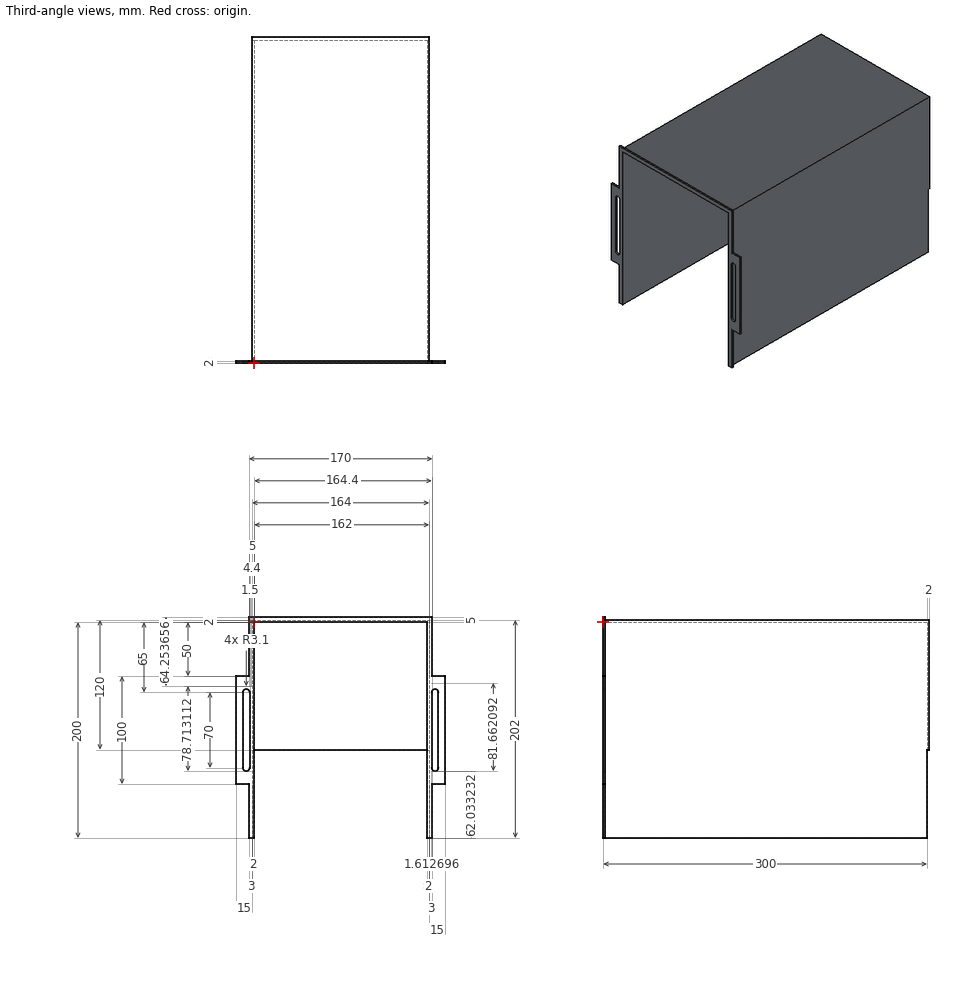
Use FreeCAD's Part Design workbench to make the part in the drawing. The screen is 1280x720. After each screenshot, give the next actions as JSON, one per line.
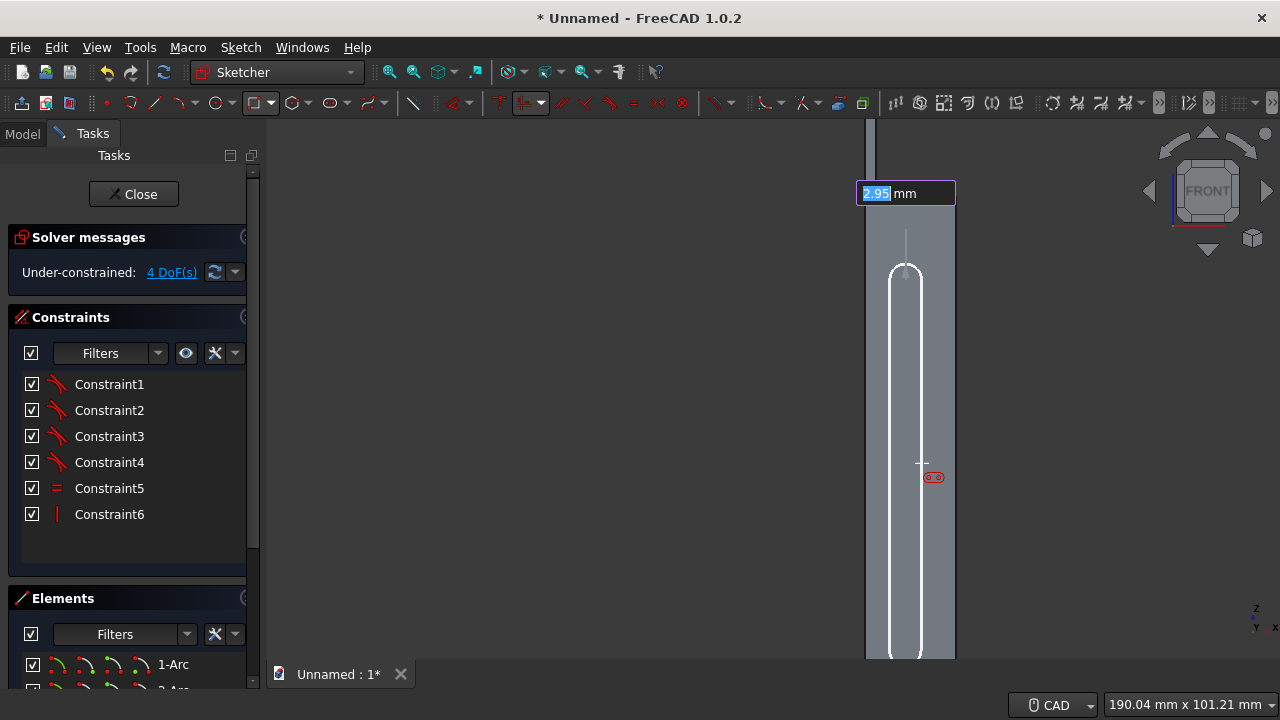
{"action": "left_click", "coordinate": [922, 463]}
{"action": "key", "text": "Escape"}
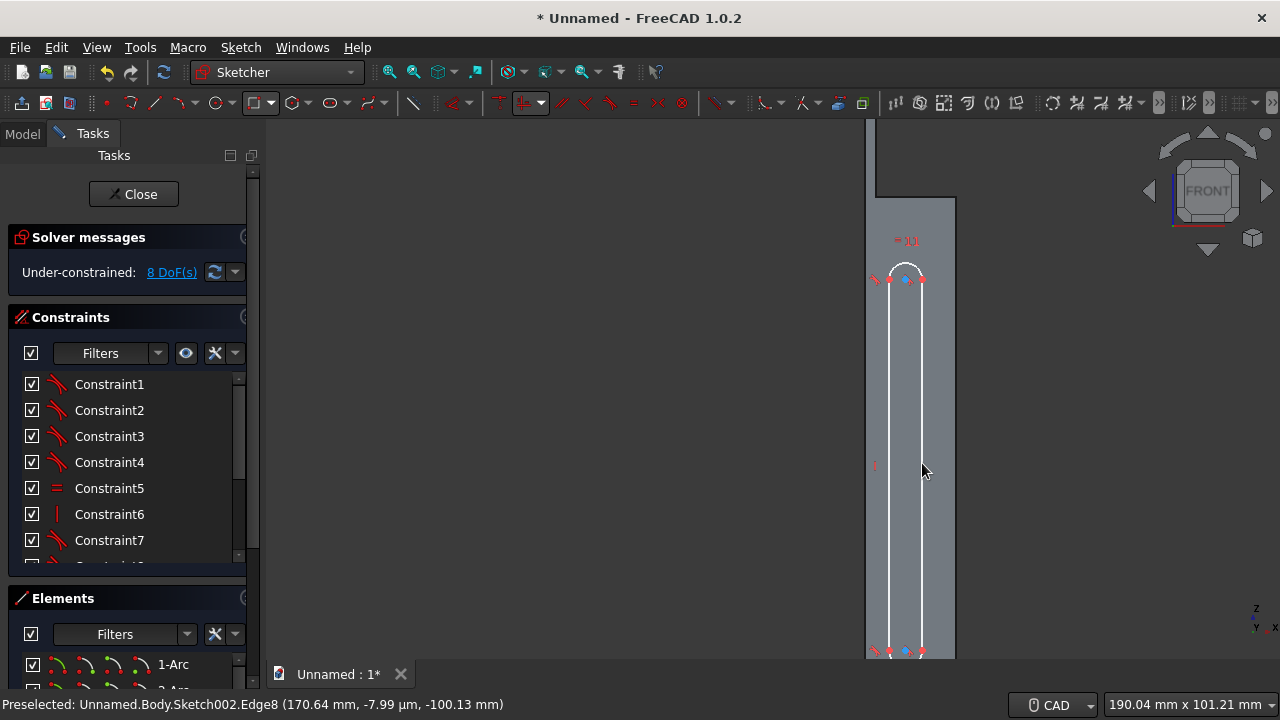
{"action": "scroll", "coordinate": [921, 463], "scroll_direction": "down", "scroll_amount": 4}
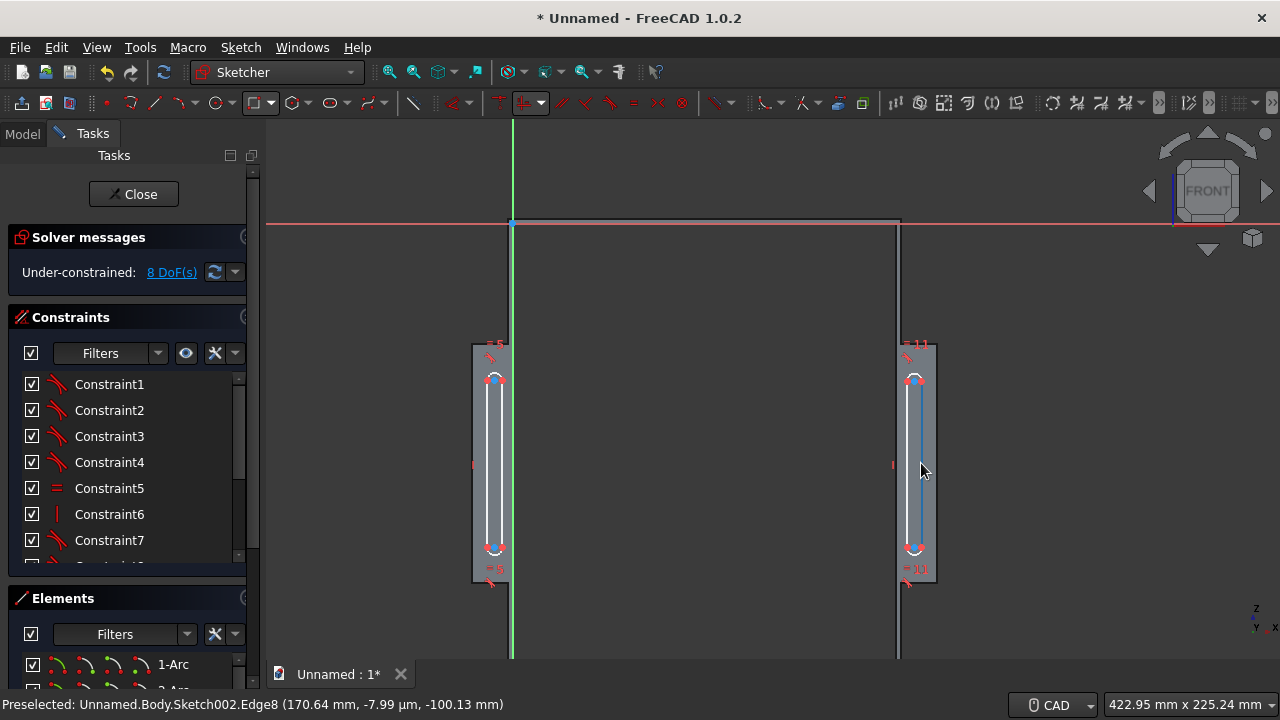
{"action": "scroll", "coordinate": [490, 554], "scroll_direction": "up", "scroll_amount": 4}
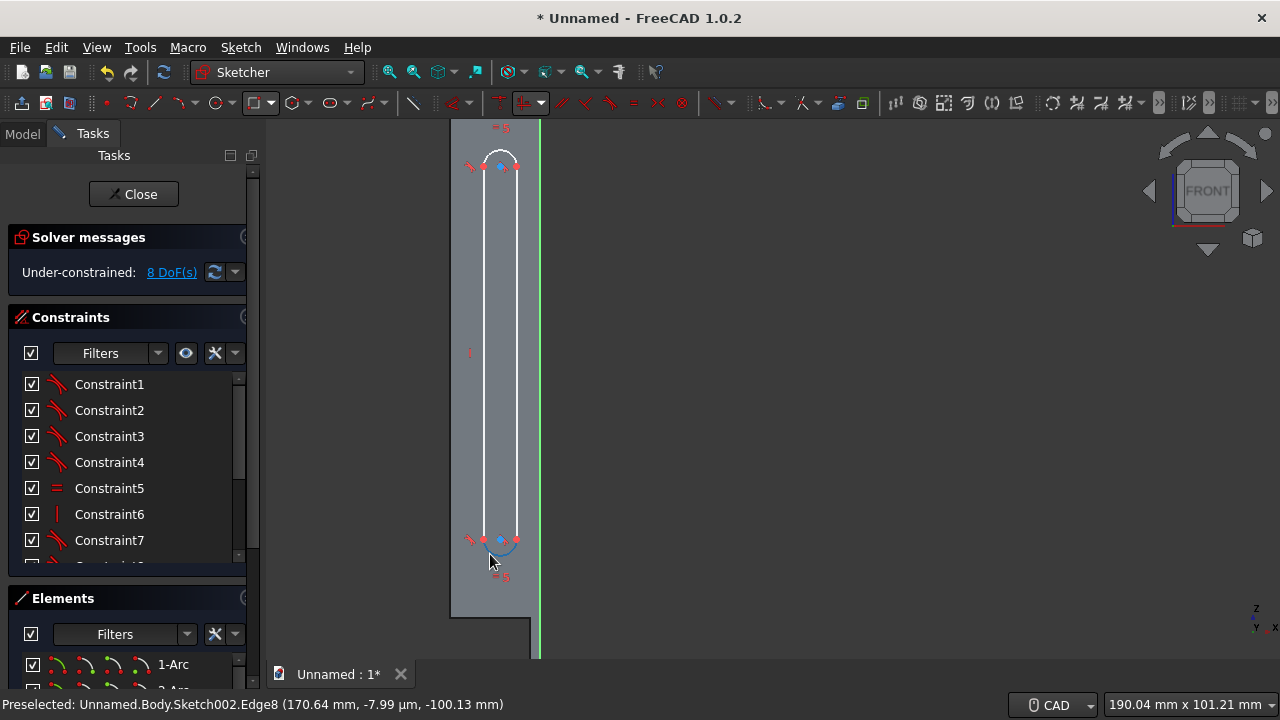
{"action": "left_click", "coordinate": [491, 553]}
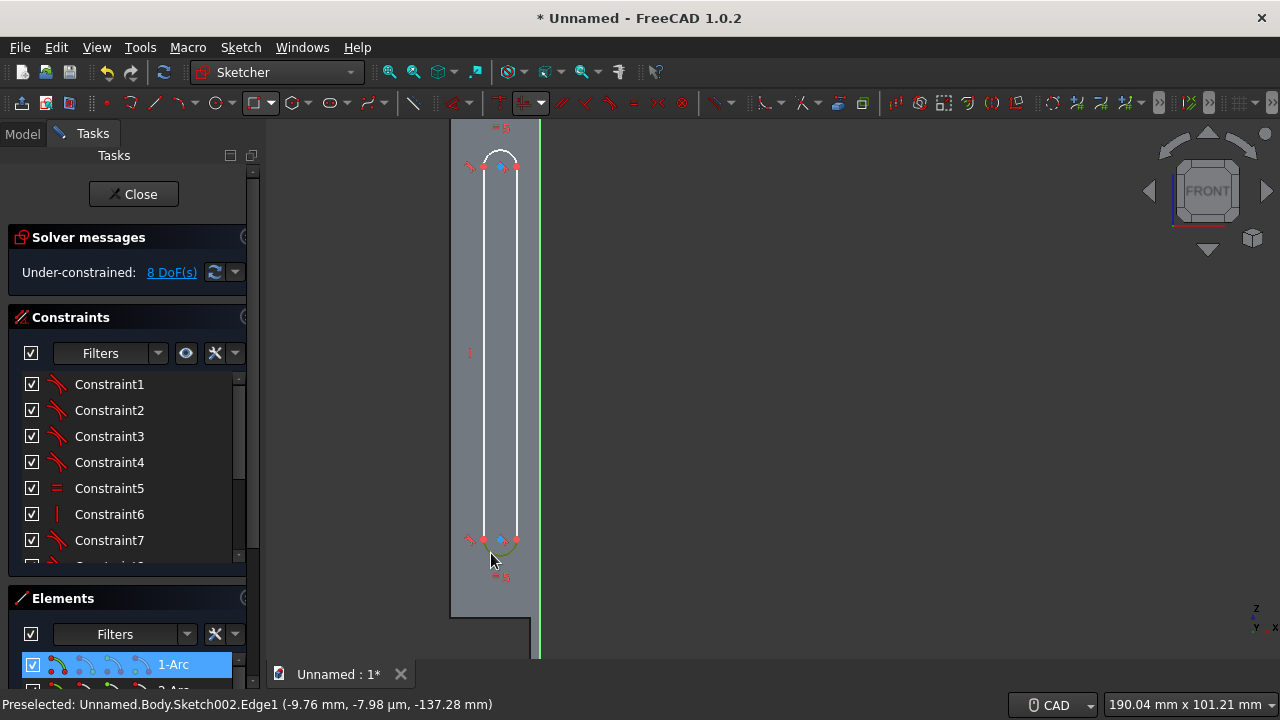
{"action": "scroll", "coordinate": [490, 554], "scroll_direction": "down", "scroll_amount": 4}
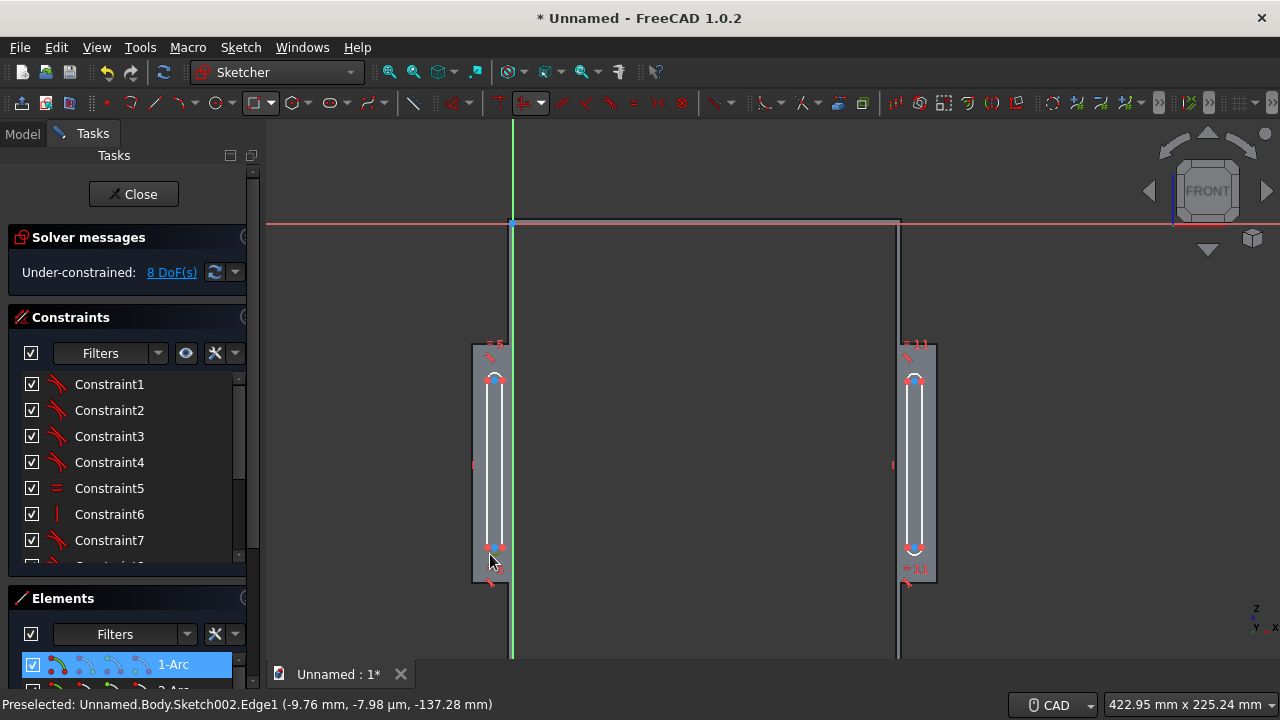
{"action": "scroll", "coordinate": [910, 554], "scroll_direction": "up", "scroll_amount": 4}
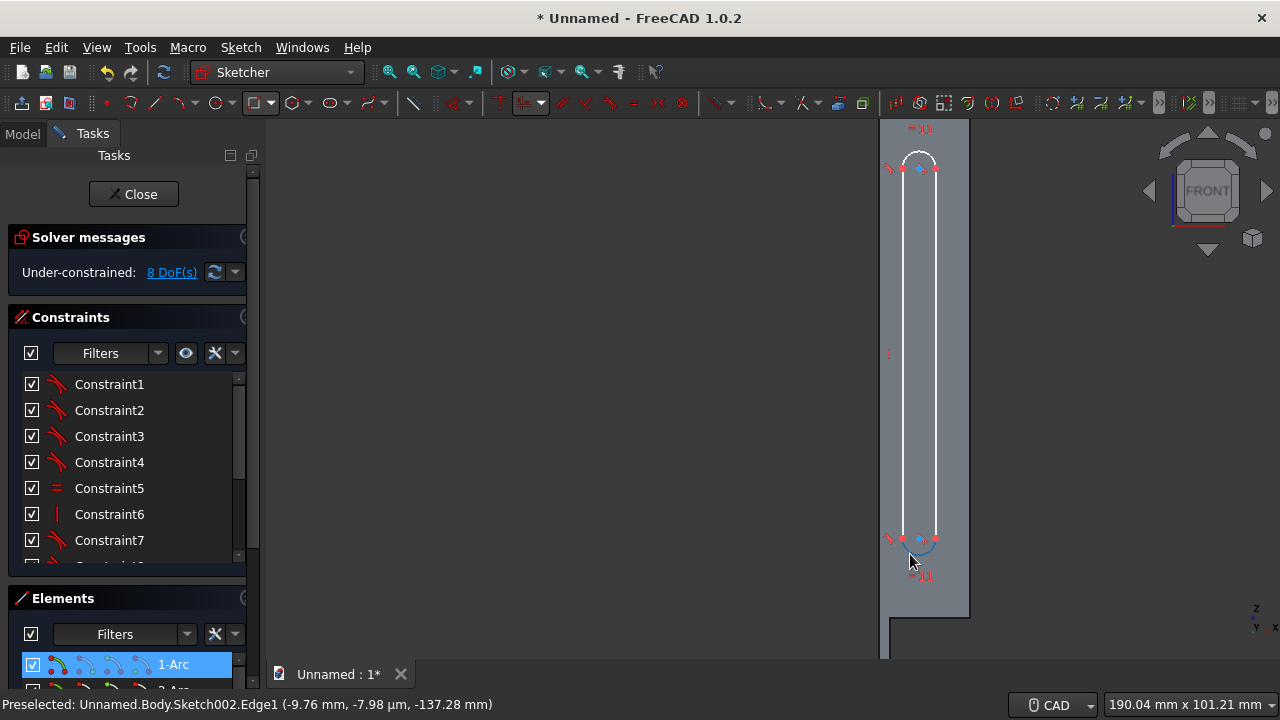
{"action": "left_click", "coordinate": [909, 552]}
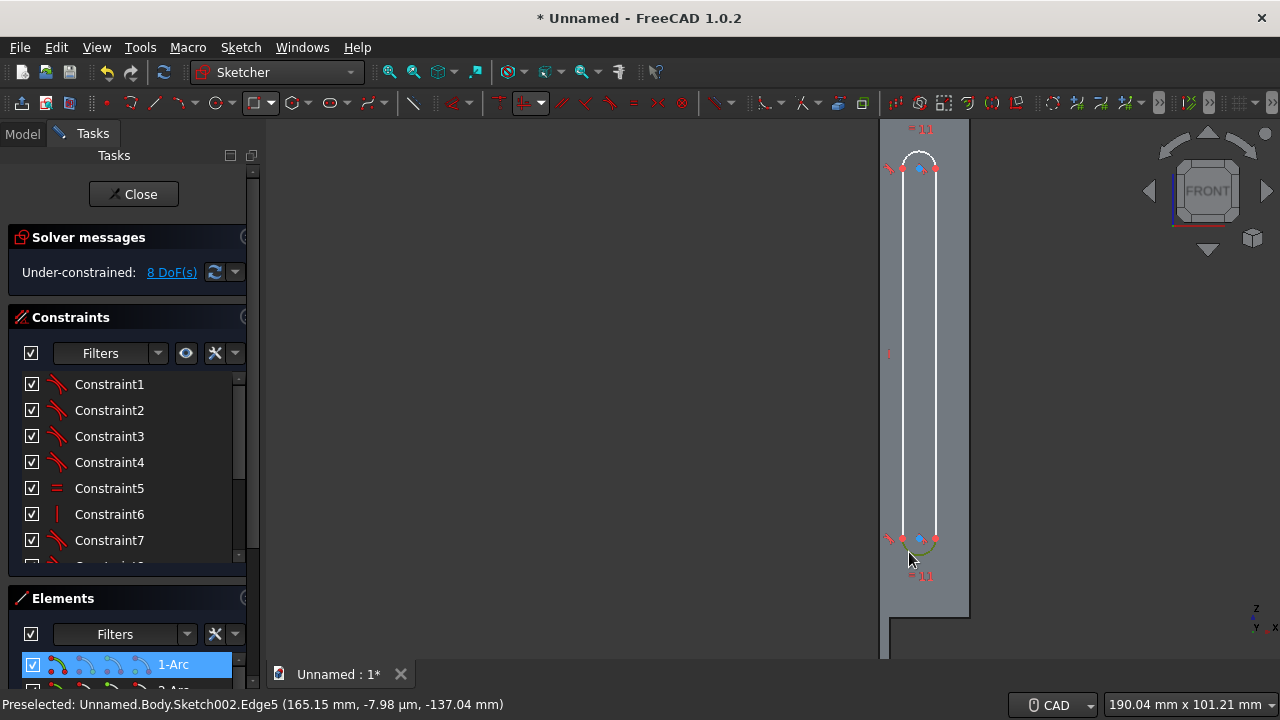
{"action": "left_click", "coordinate": [634, 104]}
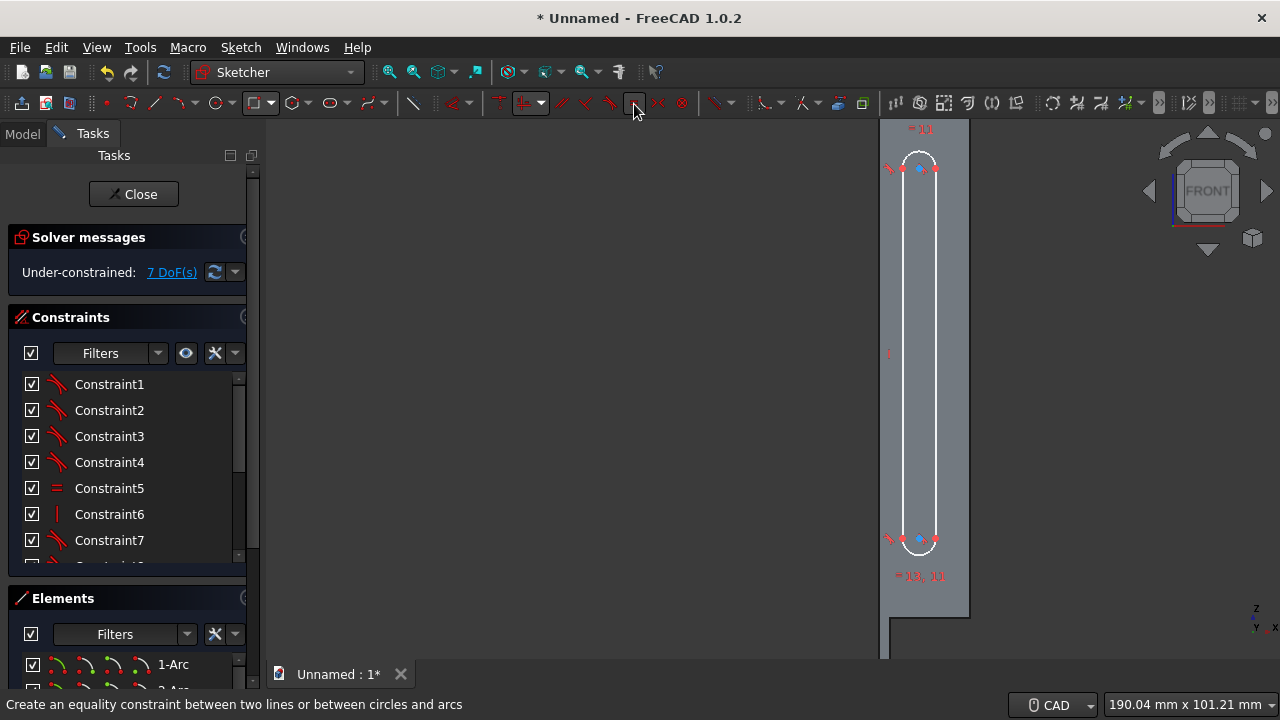
{"action": "left_click", "coordinate": [452, 104]}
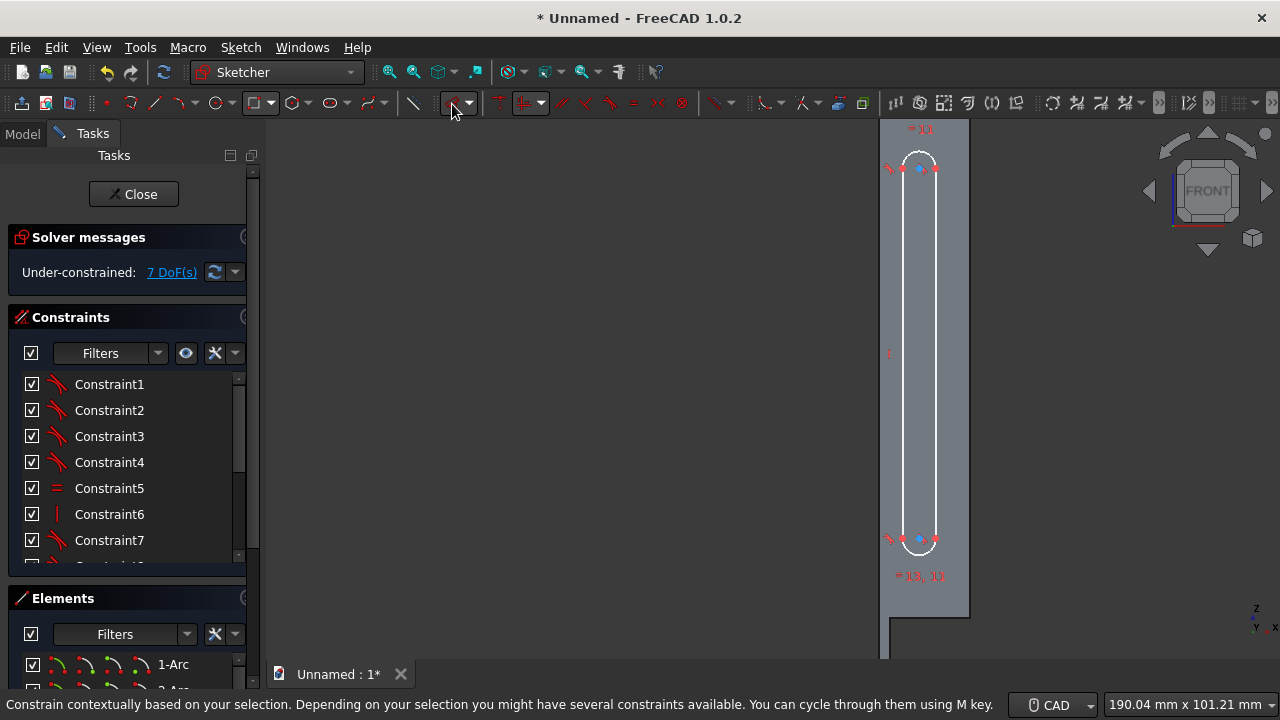
{"action": "scroll", "coordinate": [910, 554], "scroll_direction": "down", "scroll_amount": 4}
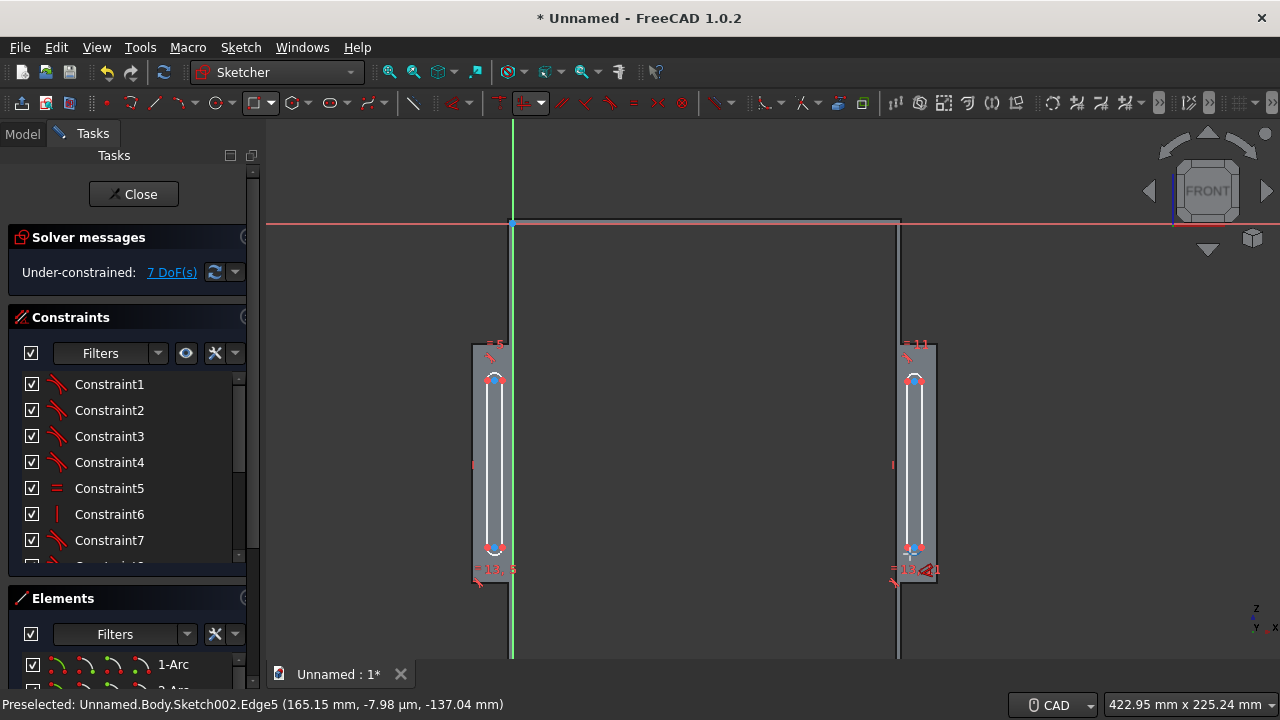
{"action": "scroll", "coordinate": [490, 554], "scroll_direction": "up", "scroll_amount": 9}